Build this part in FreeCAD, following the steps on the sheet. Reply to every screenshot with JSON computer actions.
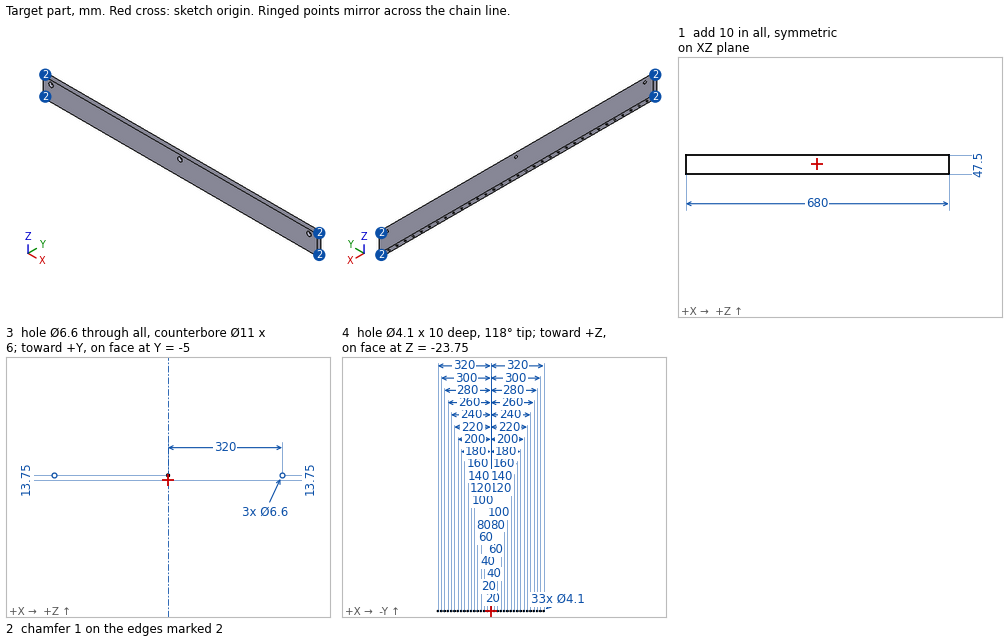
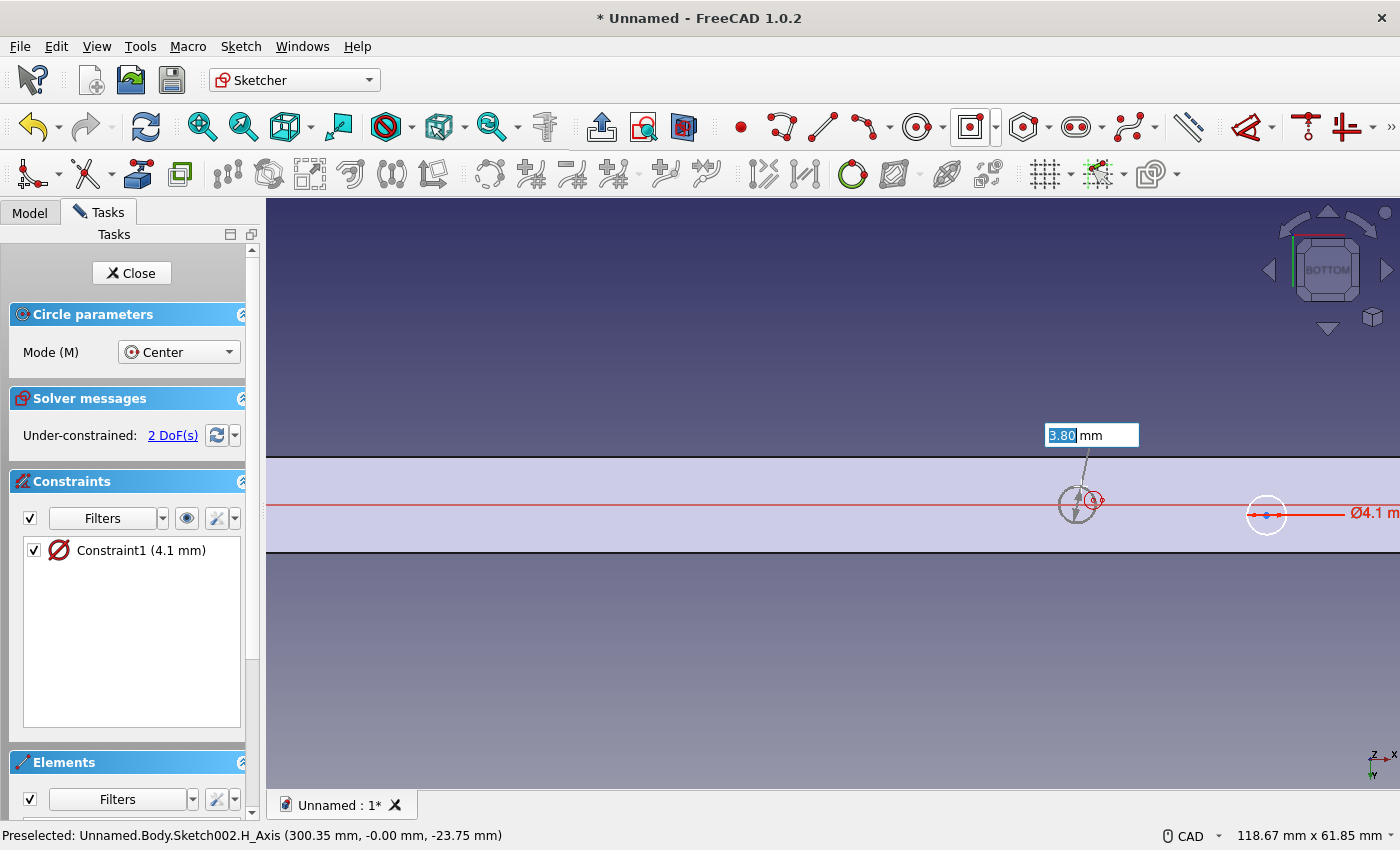
{"action": "type", "text": "4.1"}
{"action": "key", "text": "Return"}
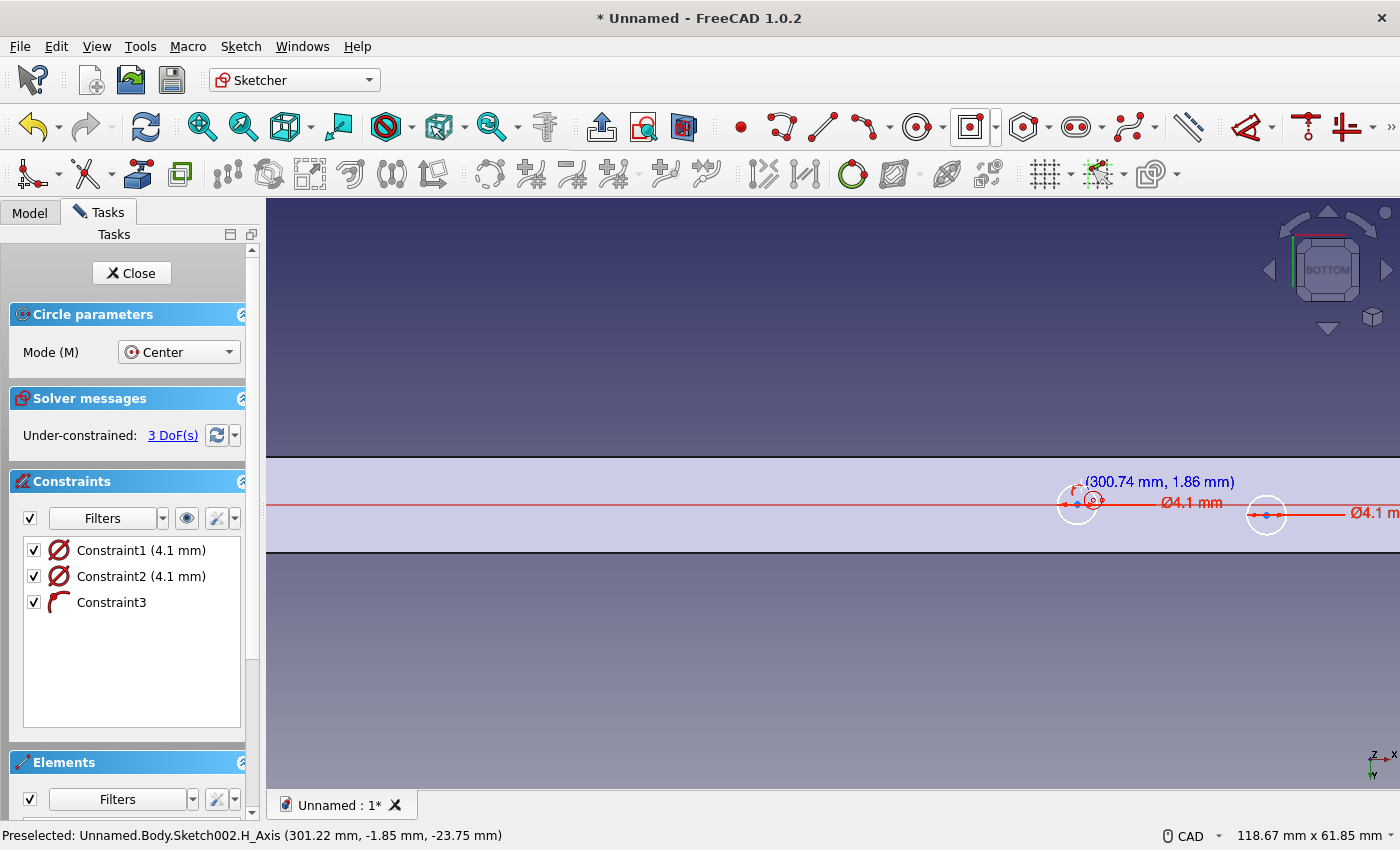
{"action": "scroll", "coordinate": [1083, 492], "scroll_direction": "down", "scroll_amount": 11}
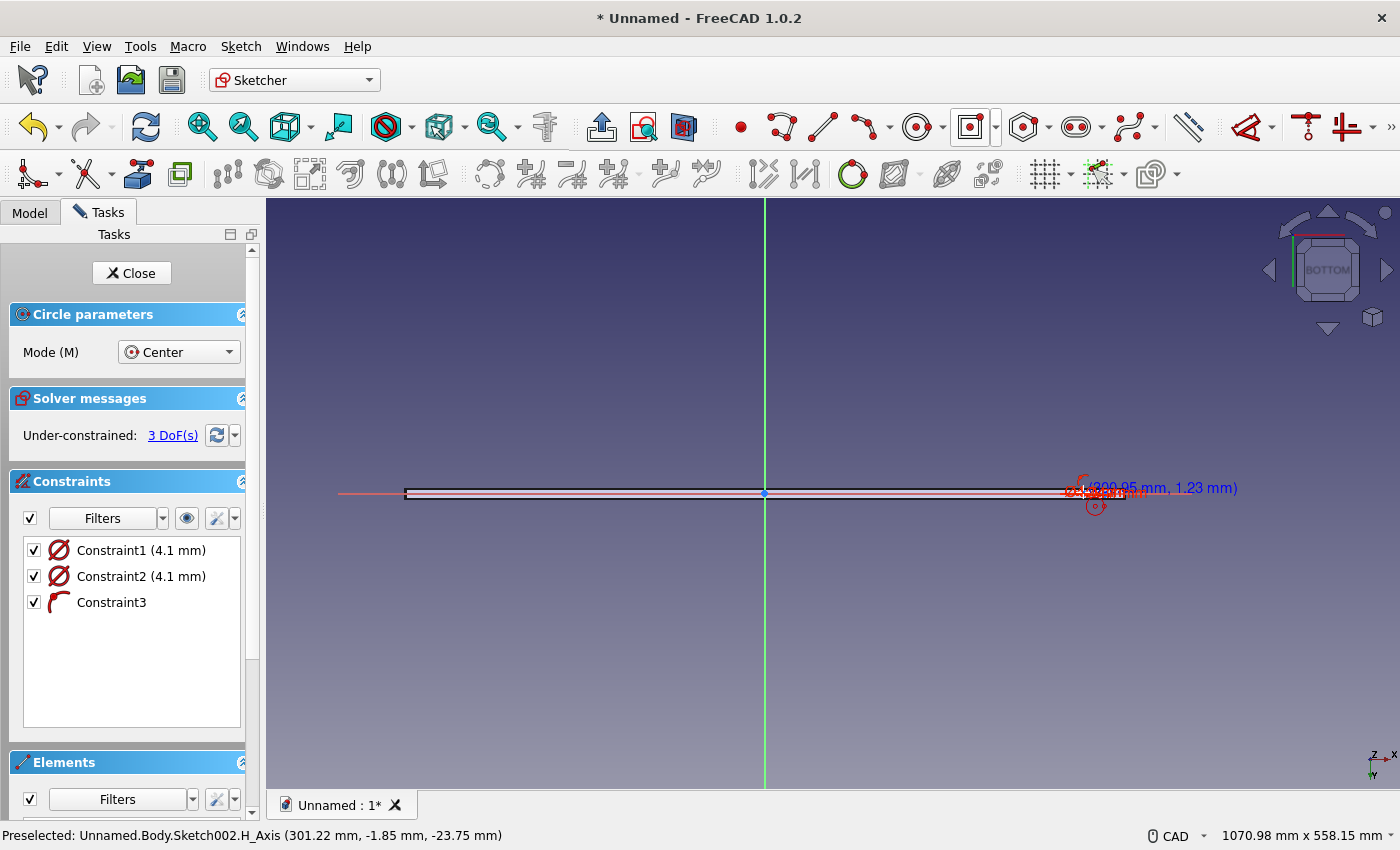
{"action": "left_click", "coordinate": [1061, 494]}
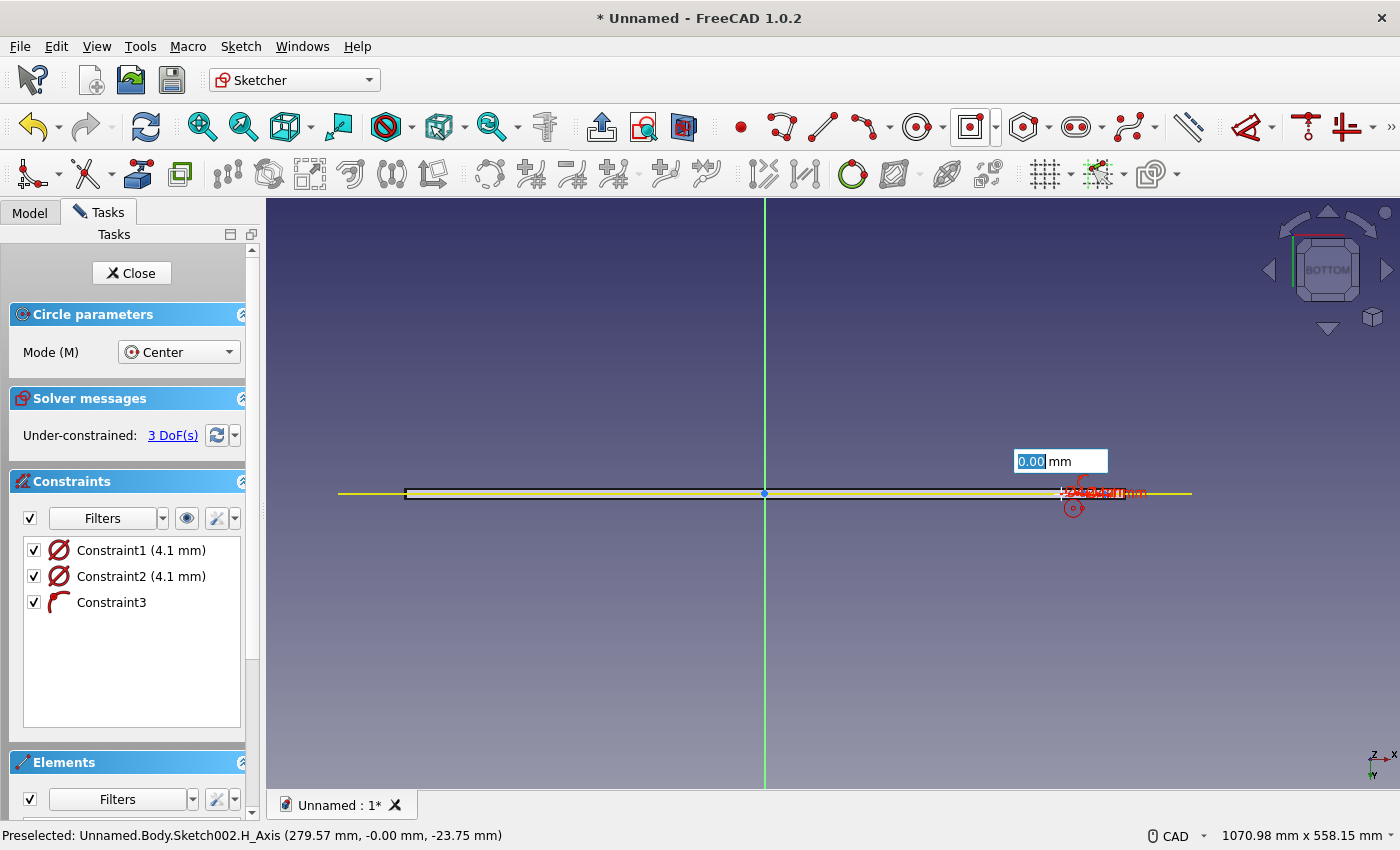
{"action": "scroll", "coordinate": [1062, 492], "scroll_direction": "up", "scroll_amount": 11}
{"action": "mouse_move", "coordinate": [1058, 486]}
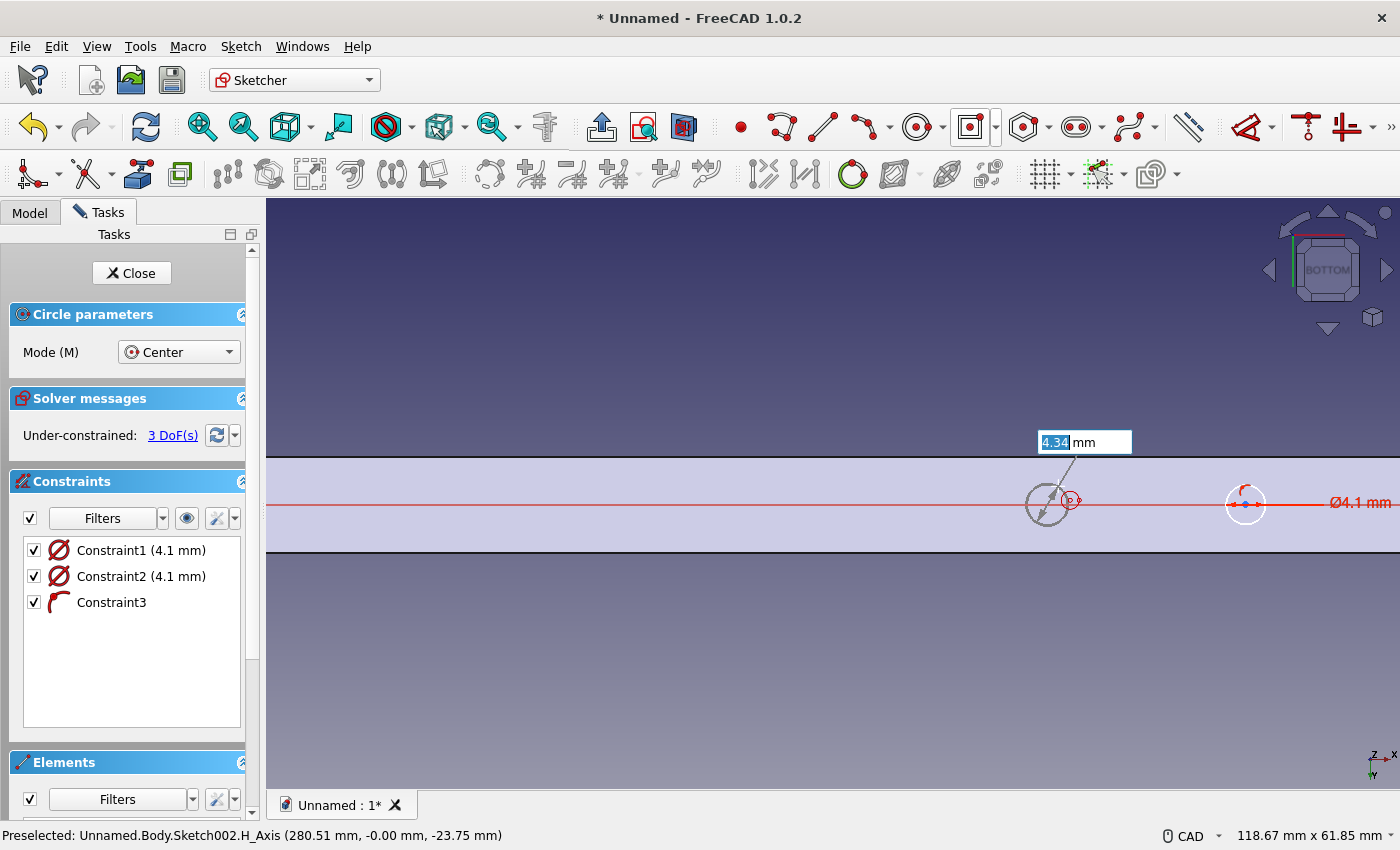
{"action": "type", "text": "4.1"}
{"action": "key", "text": "Return"}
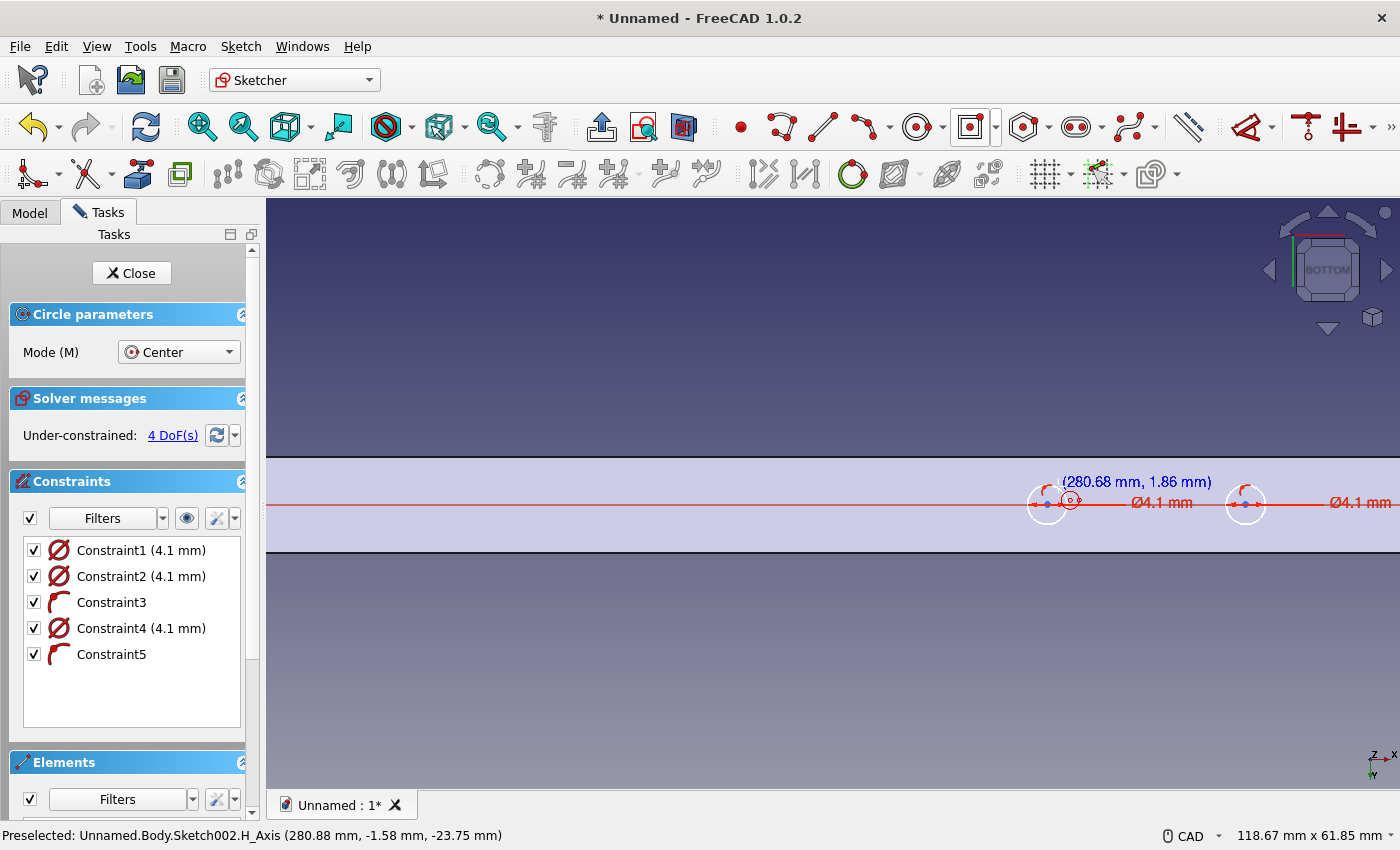
{"action": "scroll", "coordinate": [1062, 492], "scroll_direction": "down", "scroll_amount": 11}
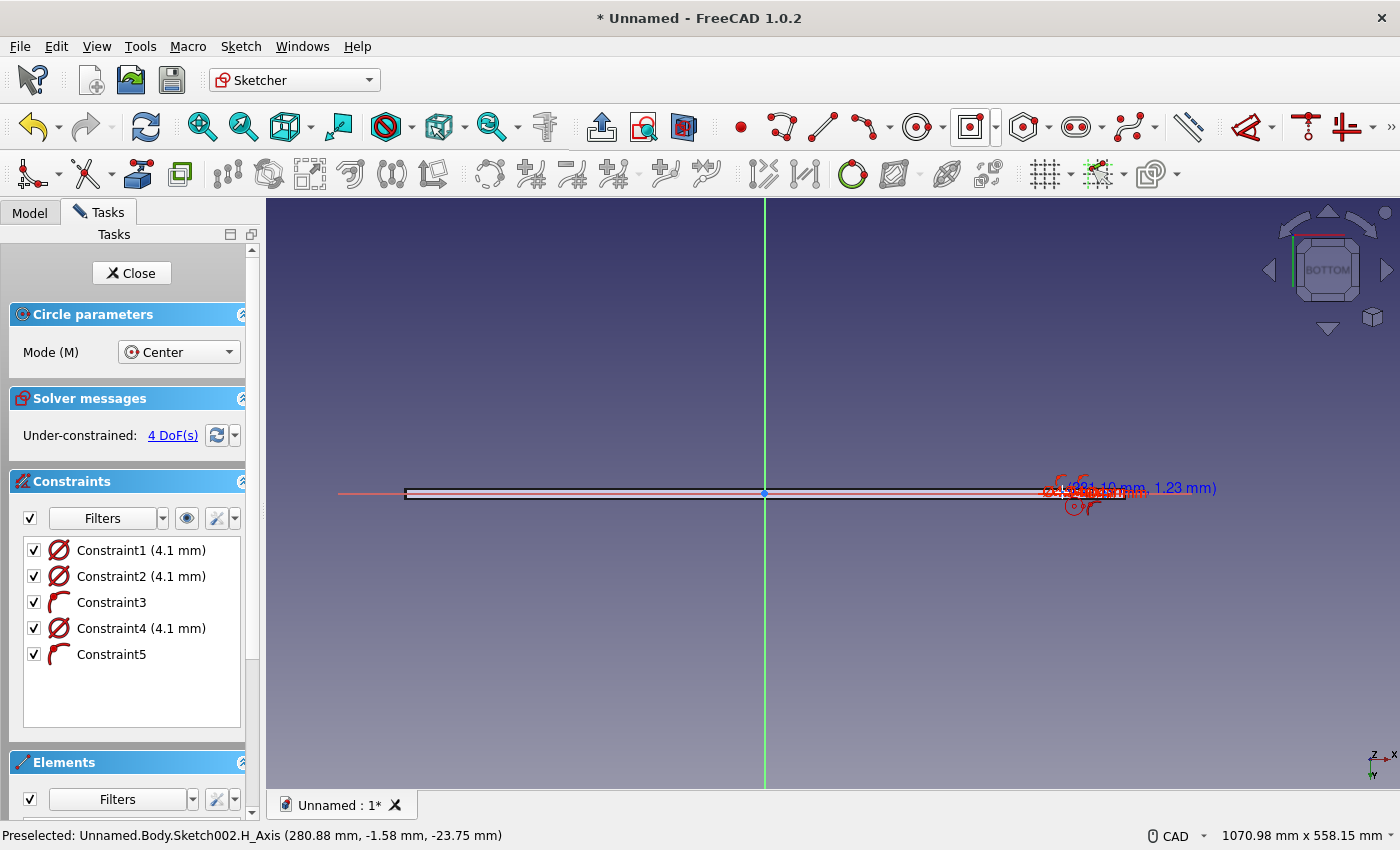
{"action": "left_click", "coordinate": [1040, 494]}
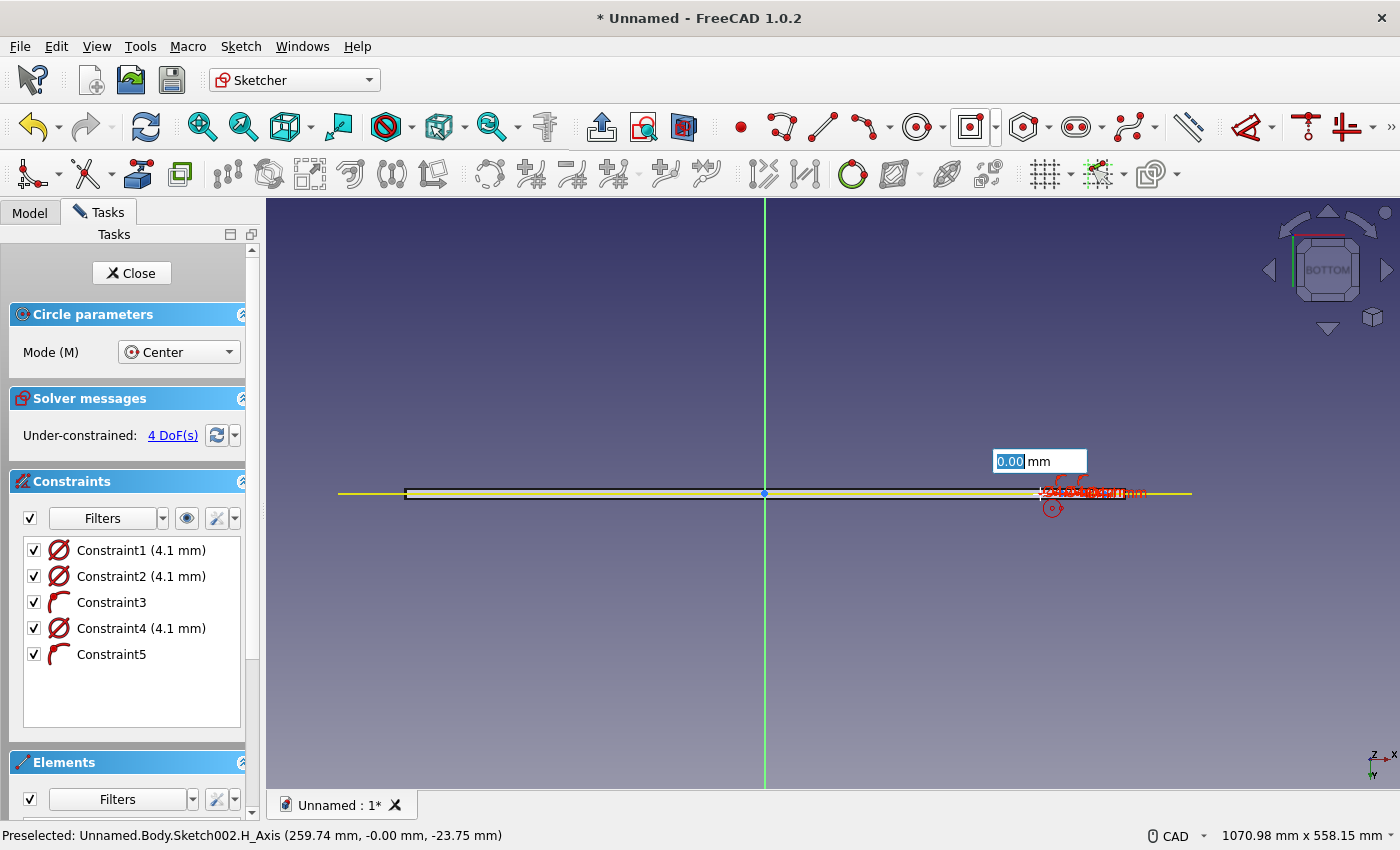
{"action": "scroll", "coordinate": [1040, 496], "scroll_direction": "up", "scroll_amount": 11}
{"action": "mouse_move", "coordinate": [1030, 491]}